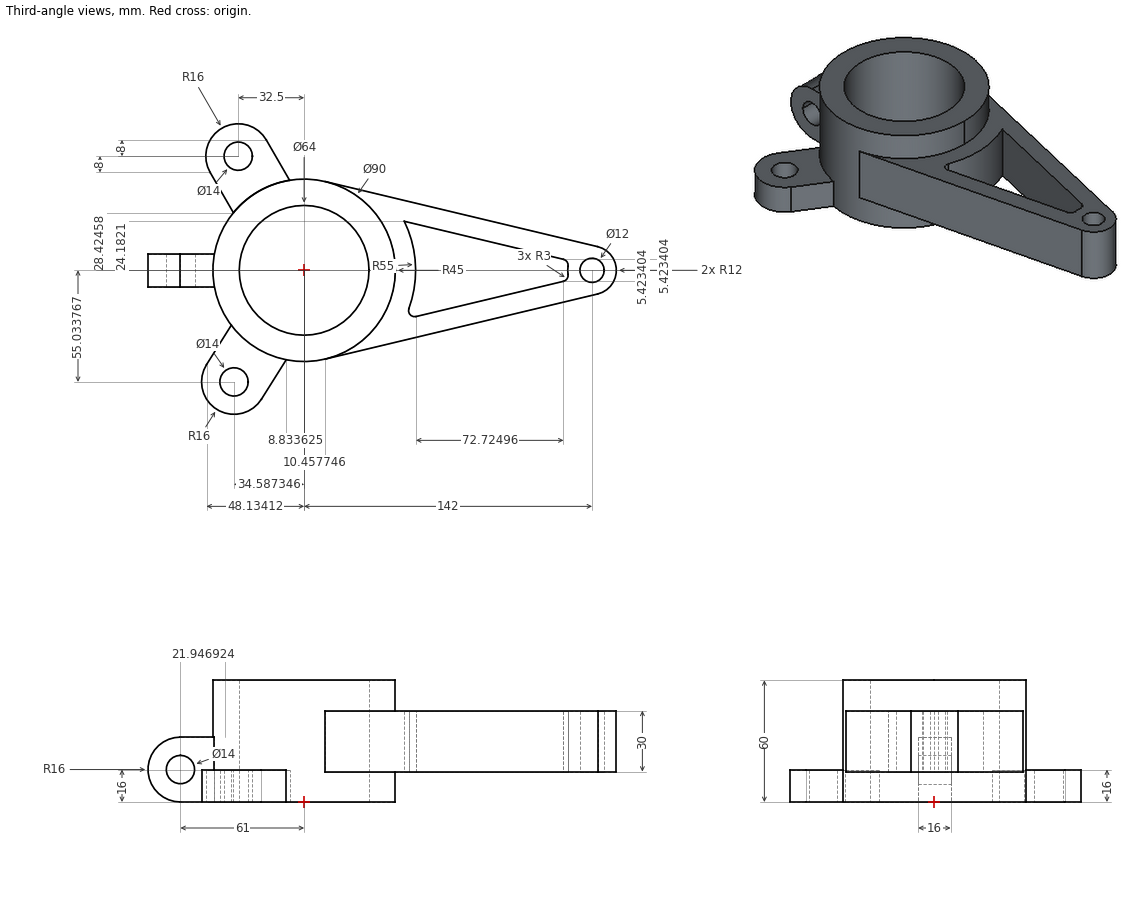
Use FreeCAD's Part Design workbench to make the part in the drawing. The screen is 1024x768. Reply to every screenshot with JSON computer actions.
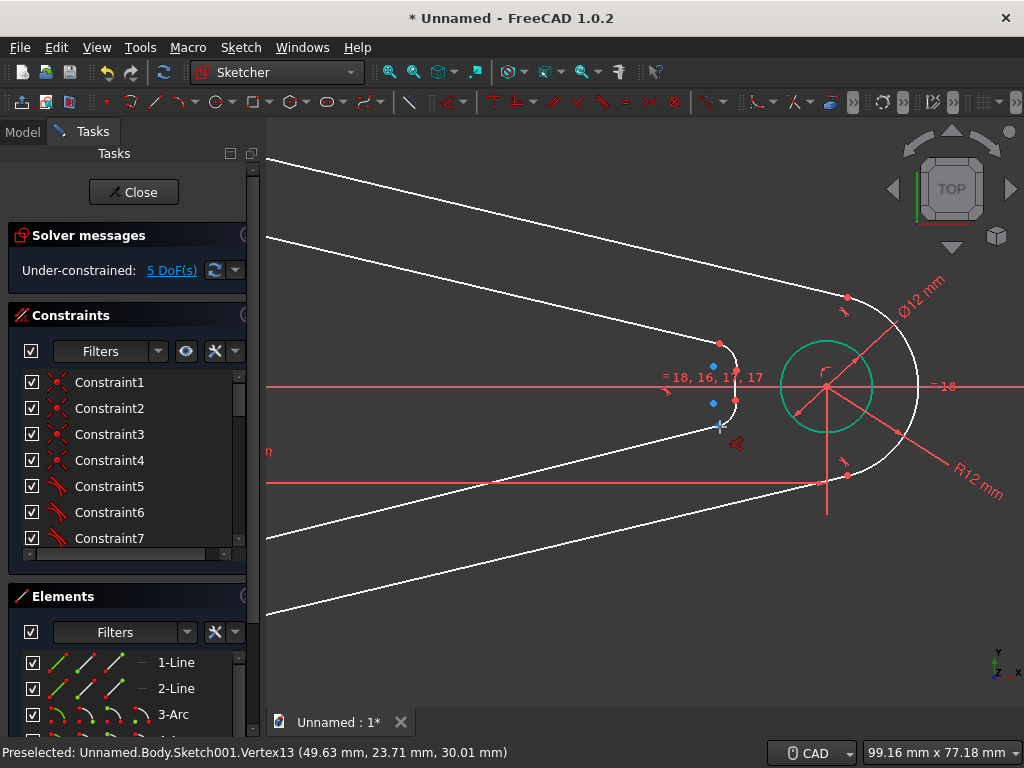
{"action": "left_click", "coordinate": [719, 426]}
{"action": "left_click", "coordinate": [753, 406]}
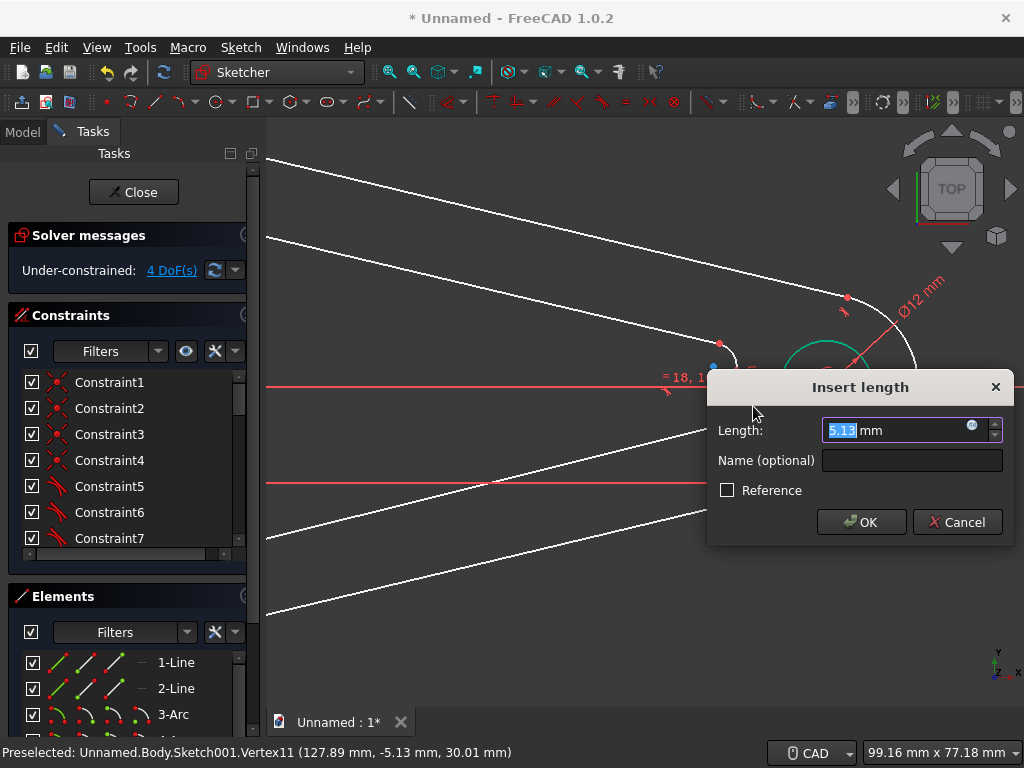
{"action": "type", "text": "5.423404"}
{"action": "key", "text": "Return"}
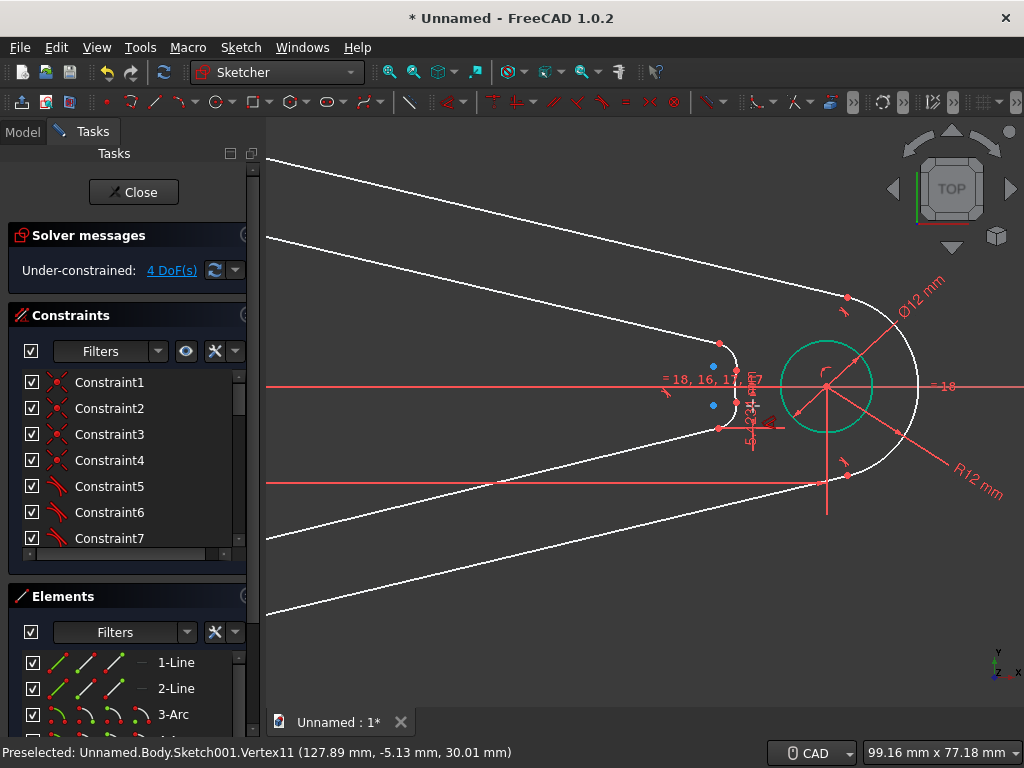
{"action": "left_click", "coordinate": [719, 344]}
{"action": "left_click", "coordinate": [753, 365]}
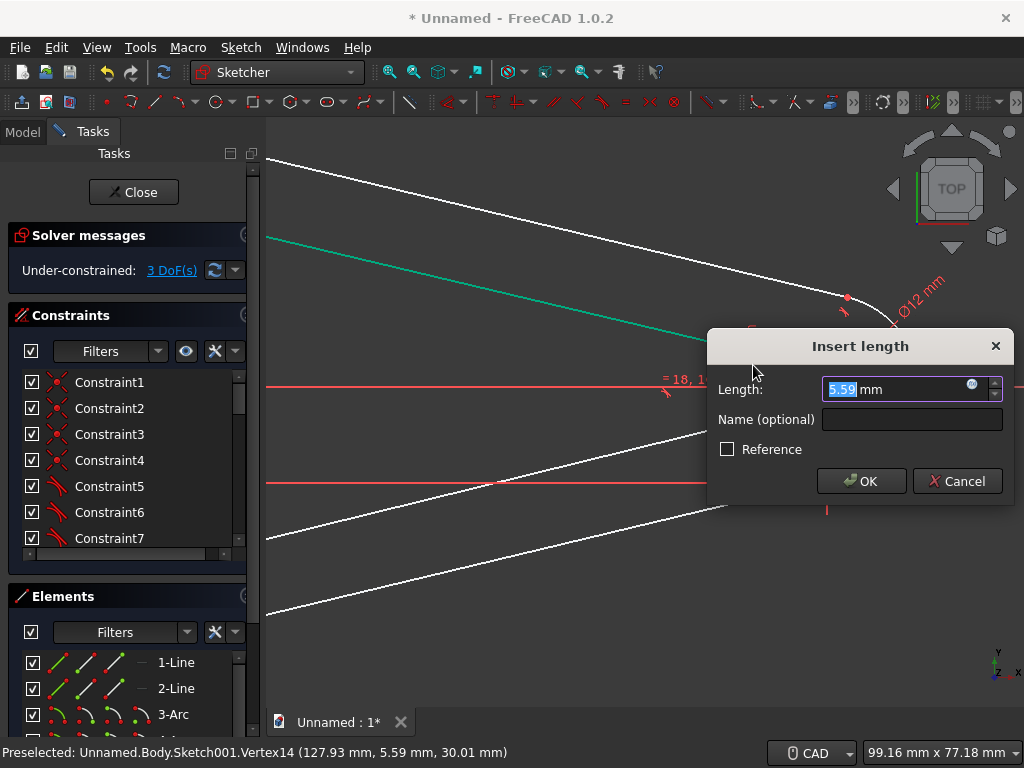
{"action": "type", "text": "5.423404"}
{"action": "key", "text": "Return"}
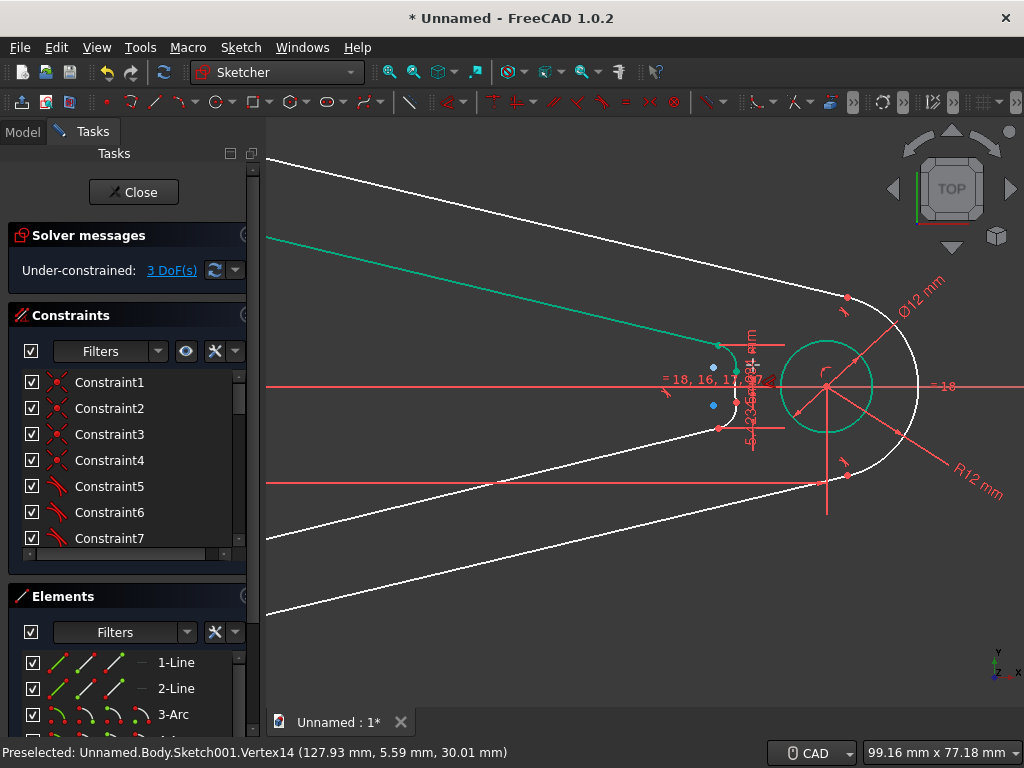
{"action": "left_click", "coordinate": [552, 469]}
{"action": "left_click", "coordinate": [506, 599]}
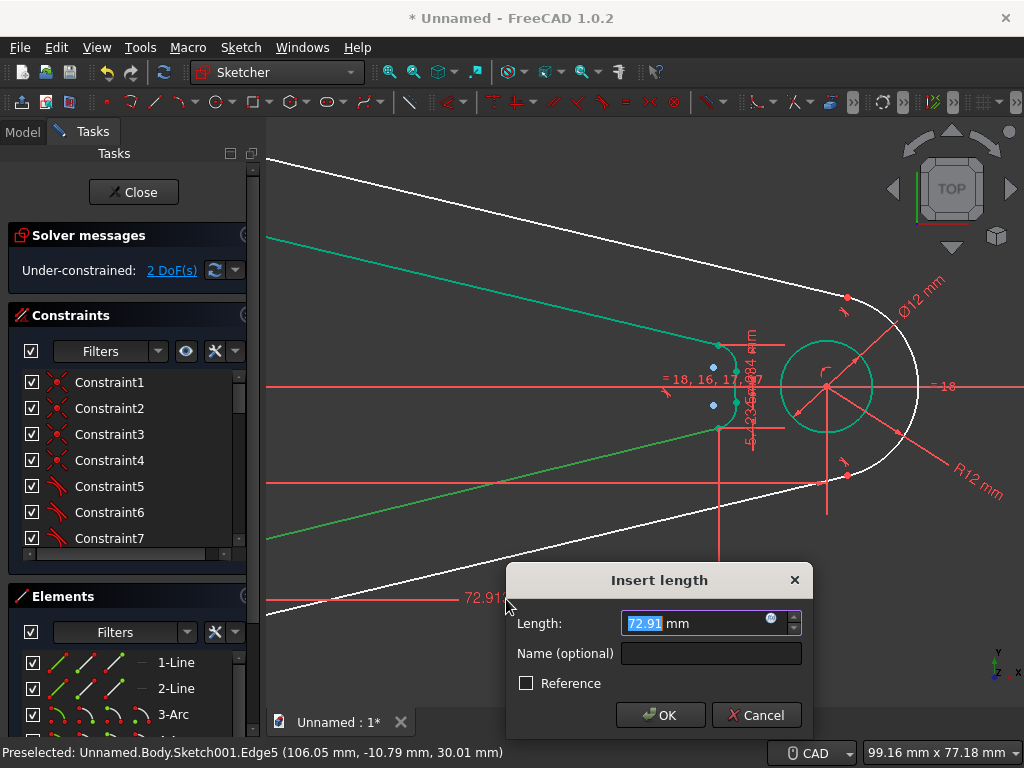
{"action": "type", "text": "72.72496"}
{"action": "key", "text": "Return"}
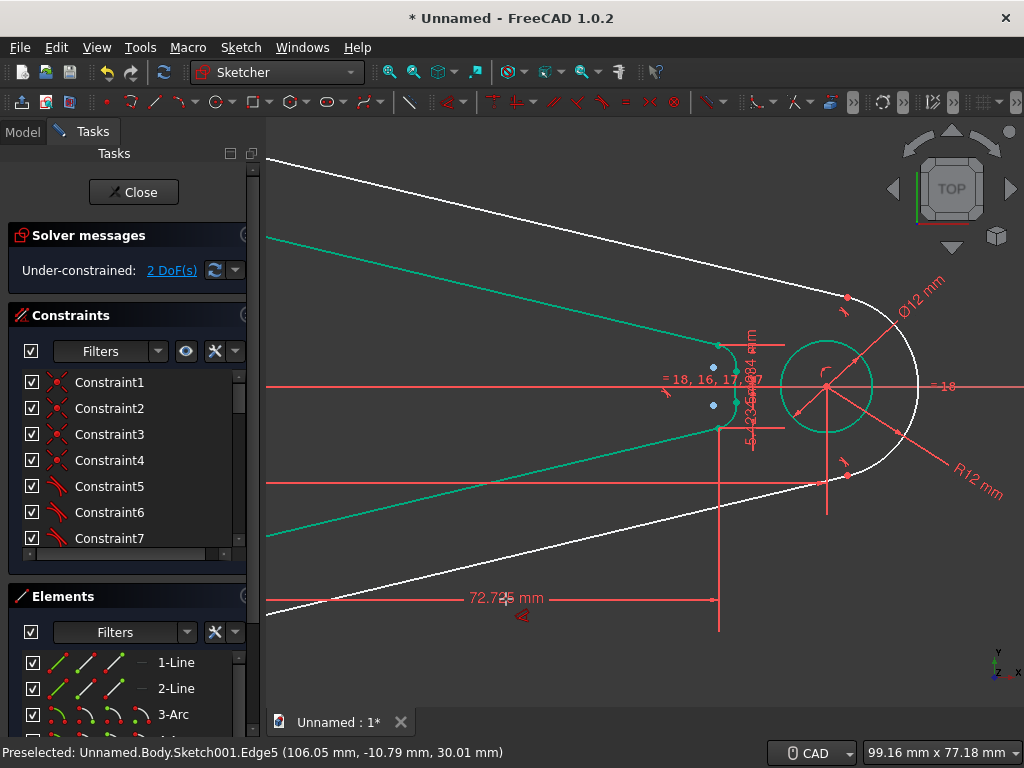
{"action": "scroll", "coordinate": [720, 427], "scroll_direction": "down", "scroll_amount": 5}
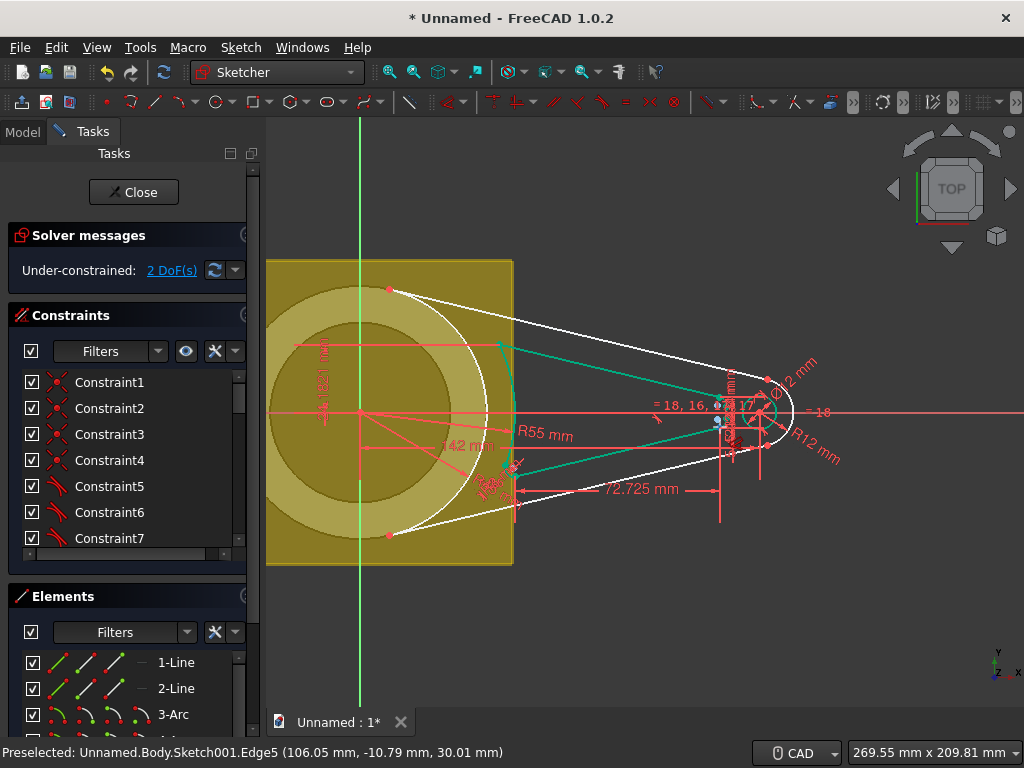
{"action": "scroll", "coordinate": [390, 536], "scroll_direction": "up", "scroll_amount": 2}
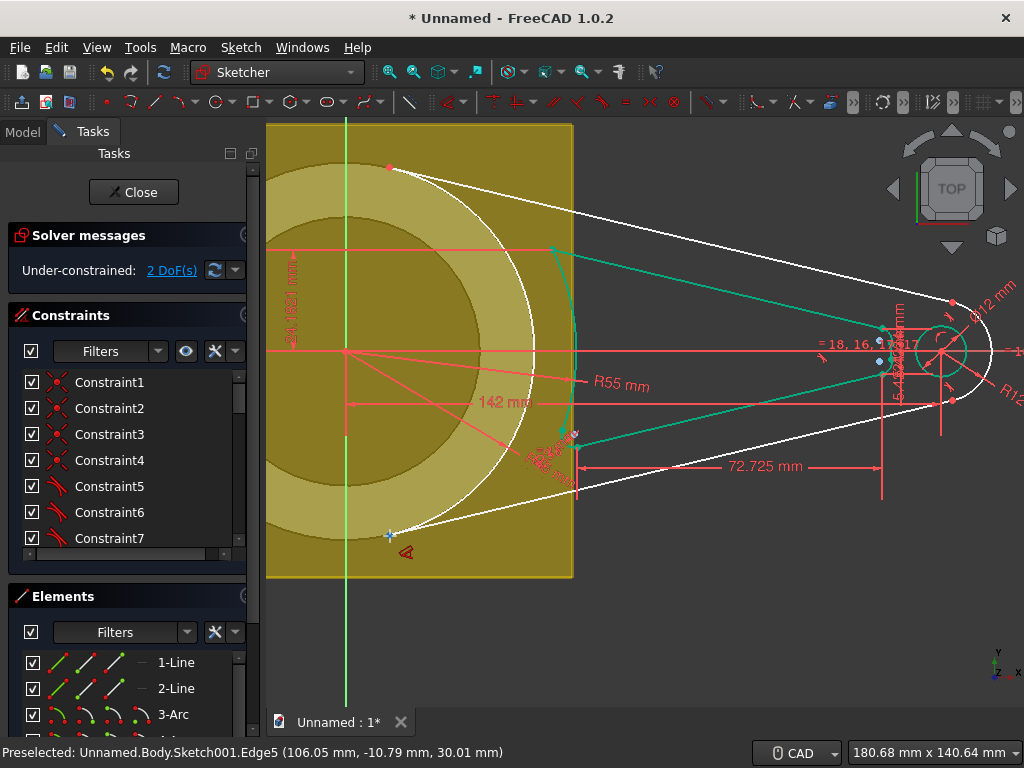
{"action": "left_click", "coordinate": [389, 535]}
{"action": "left_click", "coordinate": [367, 569]}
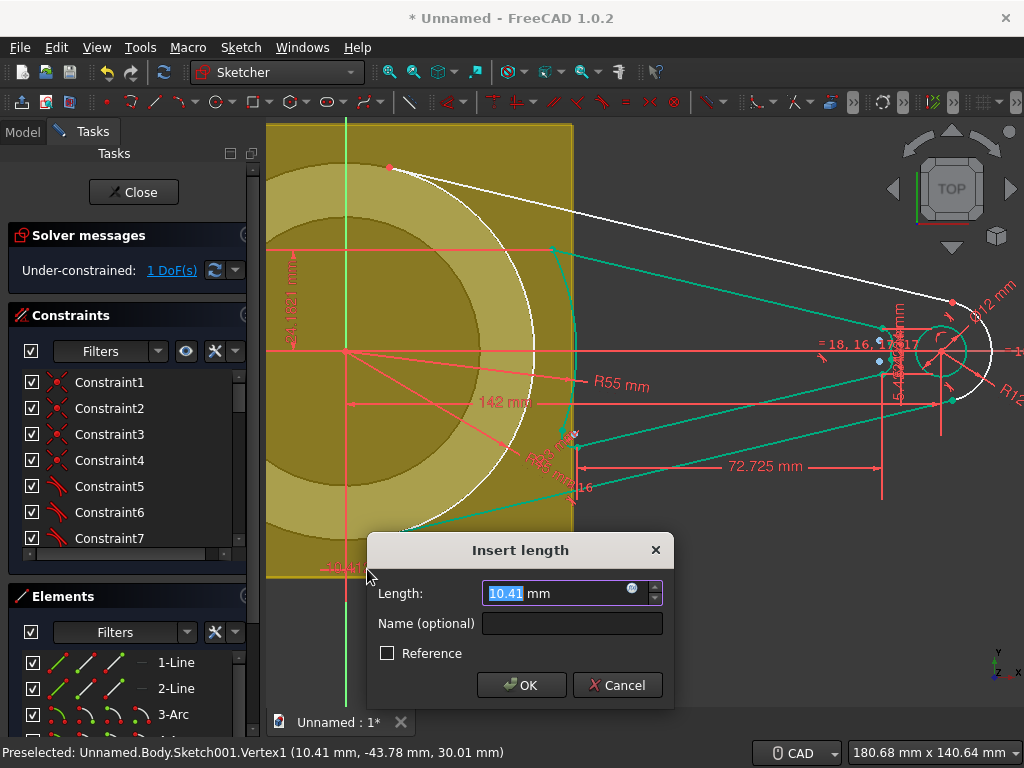
{"action": "type", "text": "10.457746"}
{"action": "key", "text": "Return"}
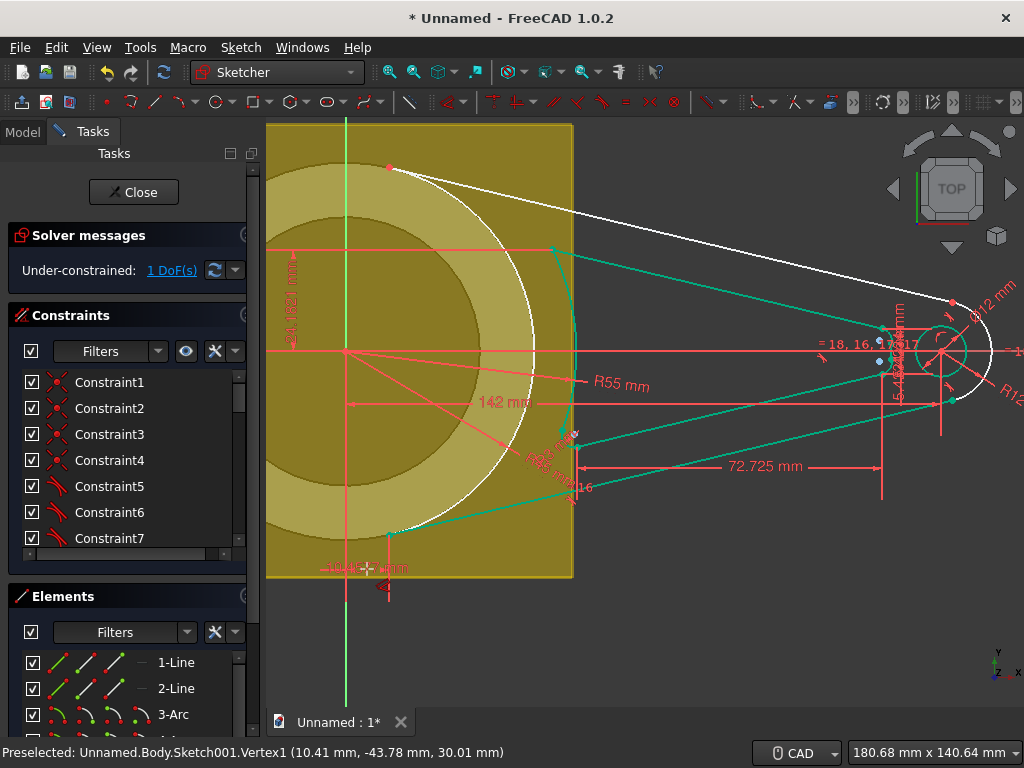
{"action": "left_click", "coordinate": [389, 168]}
{"action": "left_click", "coordinate": [367, 385]}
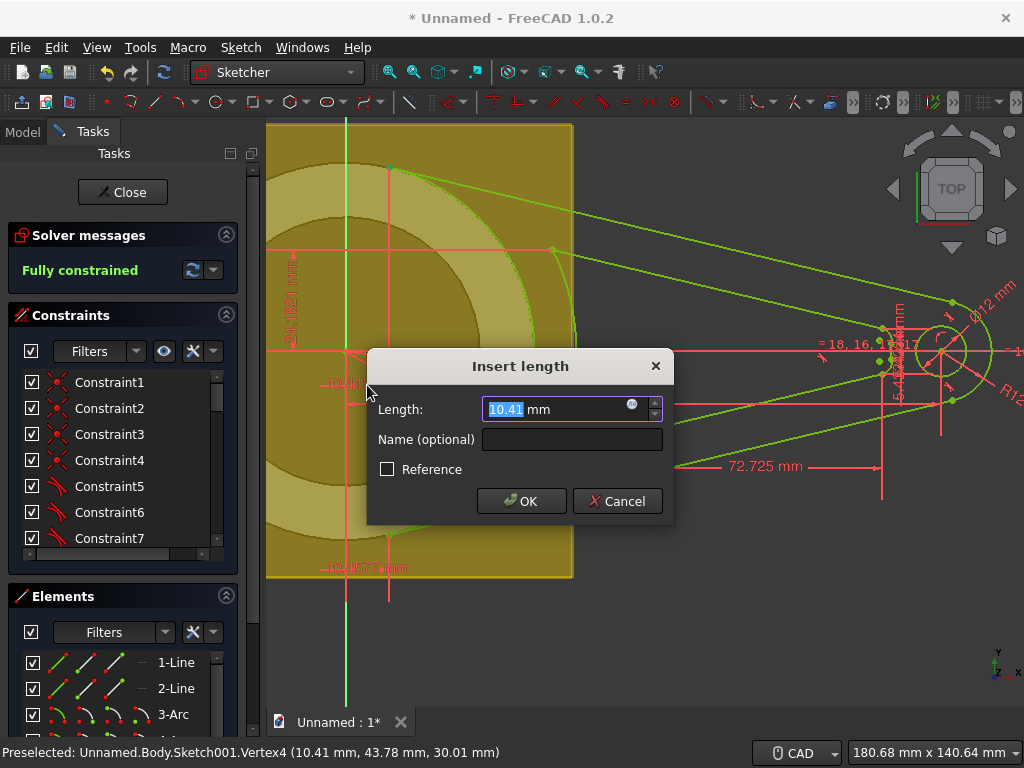
{"action": "type", "text": "10.457746"}
{"action": "key", "text": "Return"}
{"action": "key", "text": "Escape"}